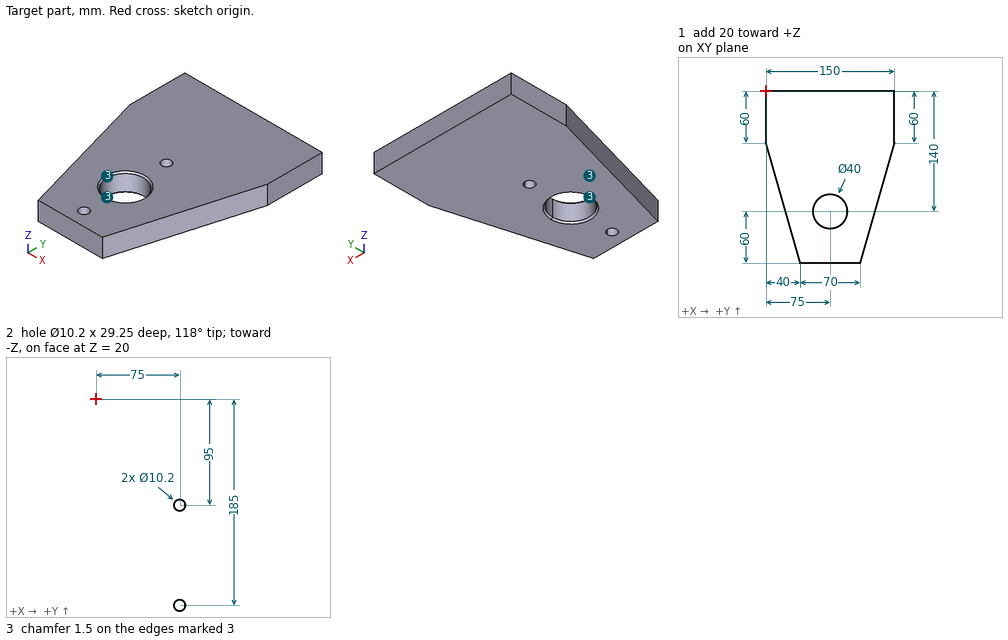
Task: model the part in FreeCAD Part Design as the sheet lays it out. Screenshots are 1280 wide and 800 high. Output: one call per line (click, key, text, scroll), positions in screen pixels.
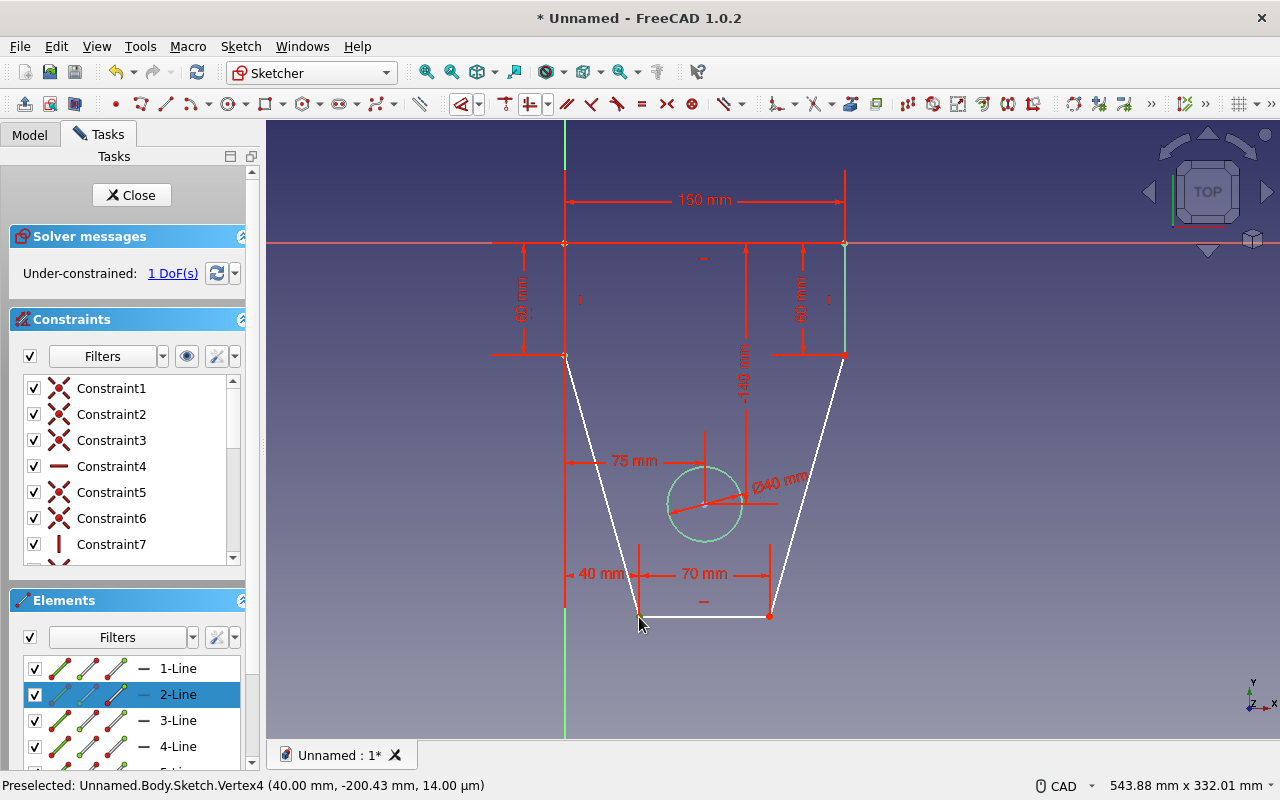
click(705, 504)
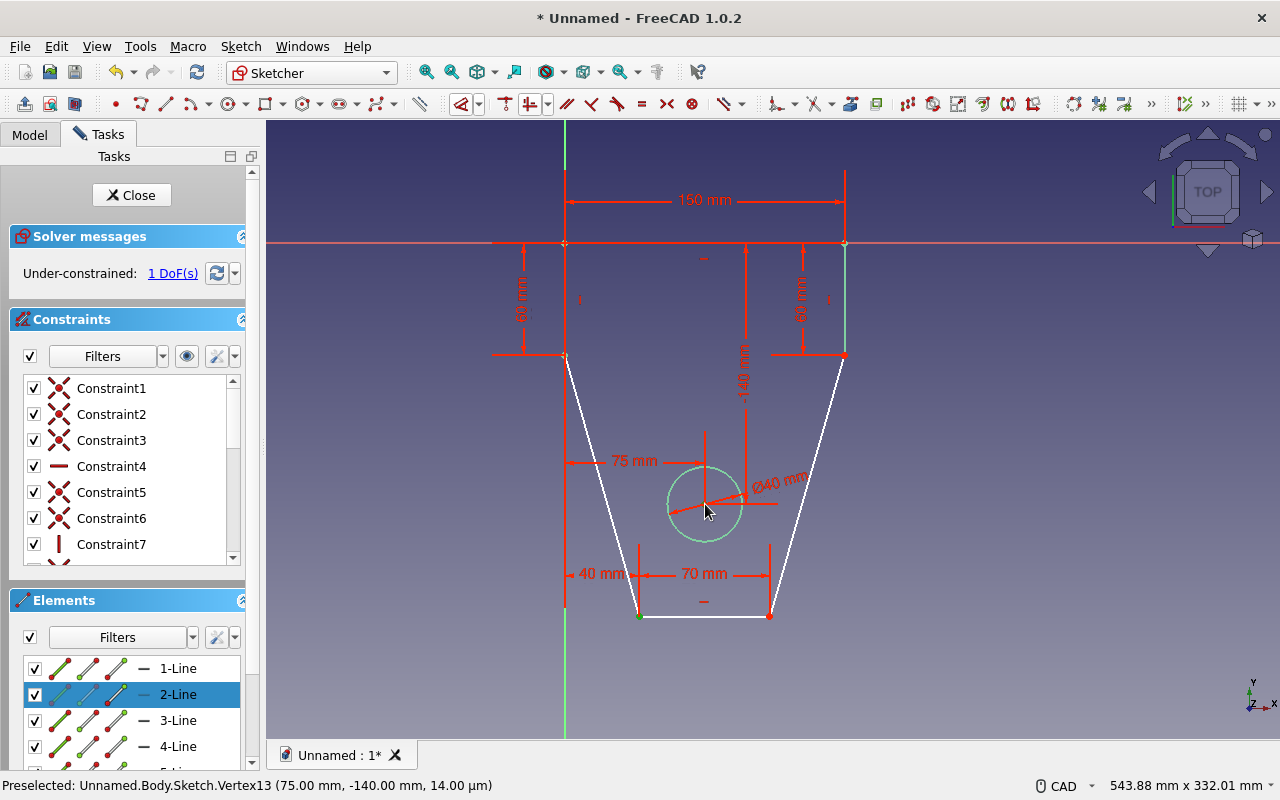
click(478, 104)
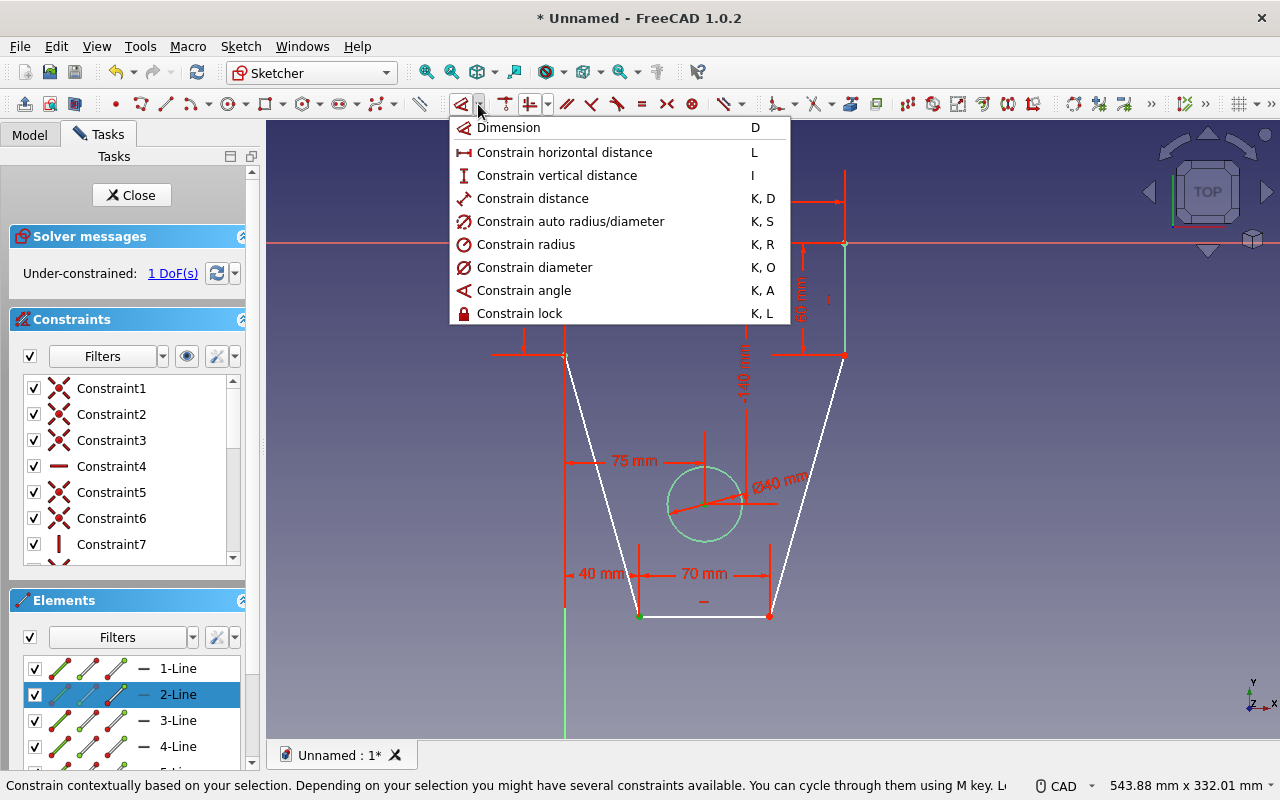
click(620, 176)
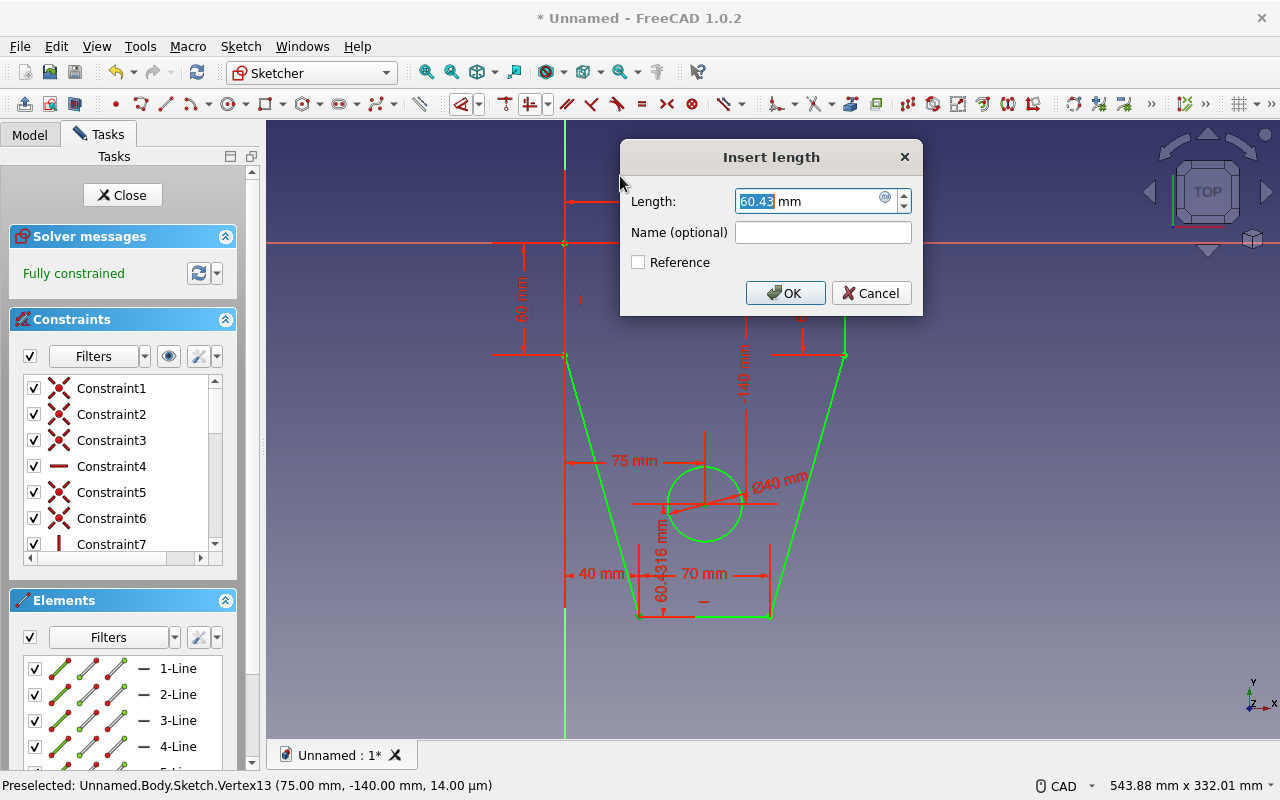
text(60)
key(Return)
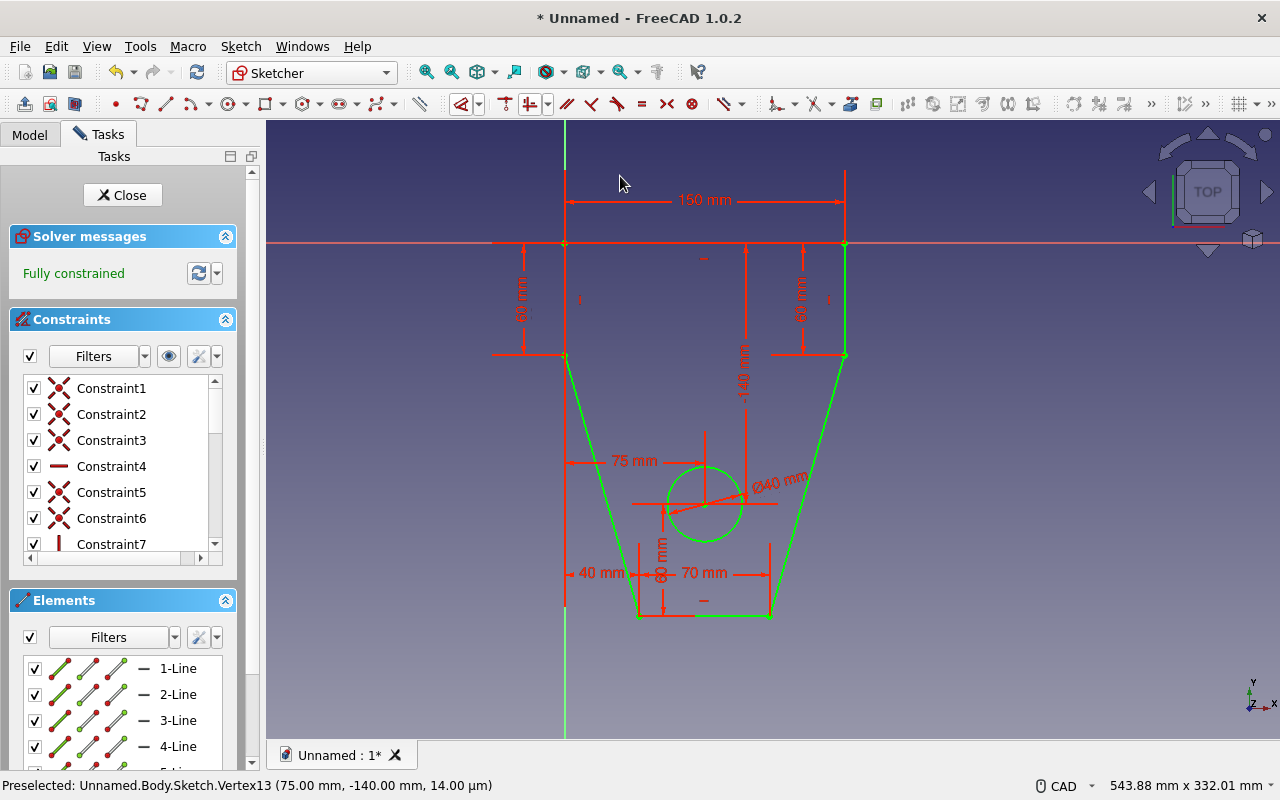
click(123, 195)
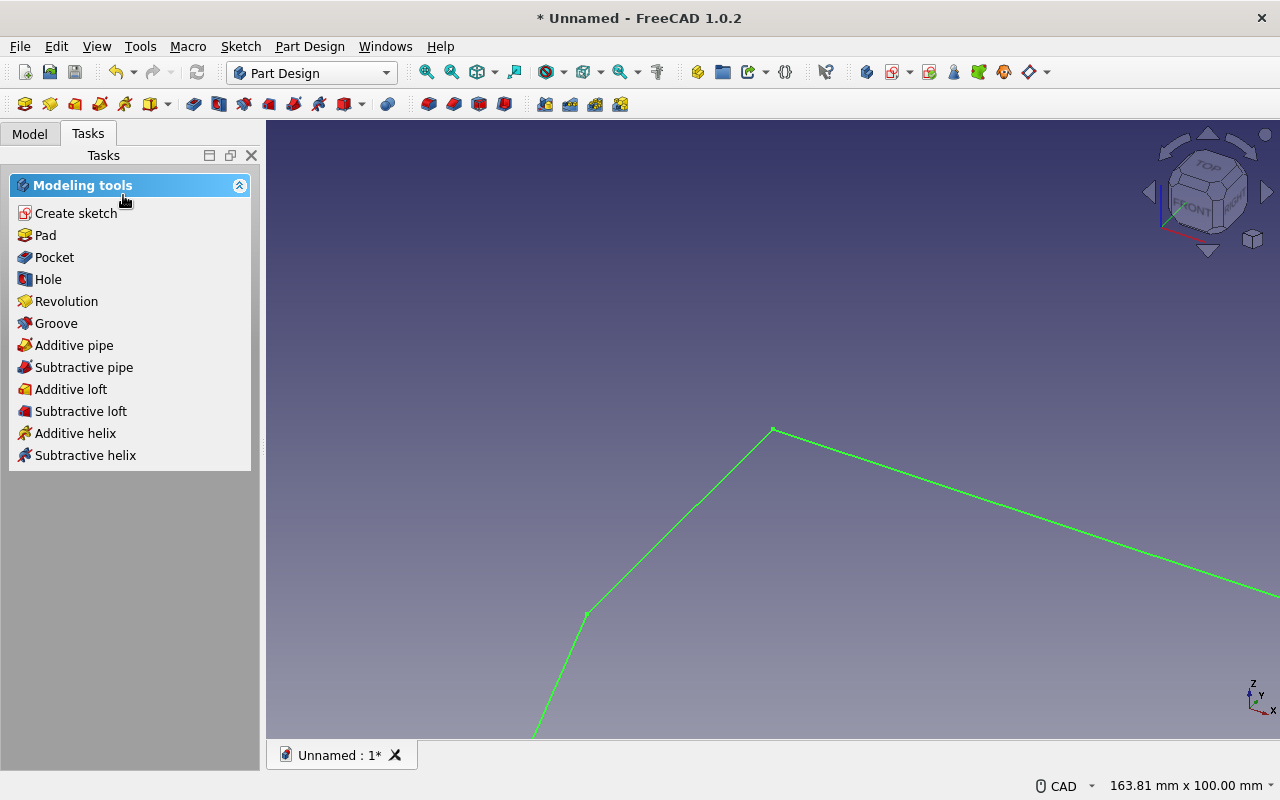
click(25, 104)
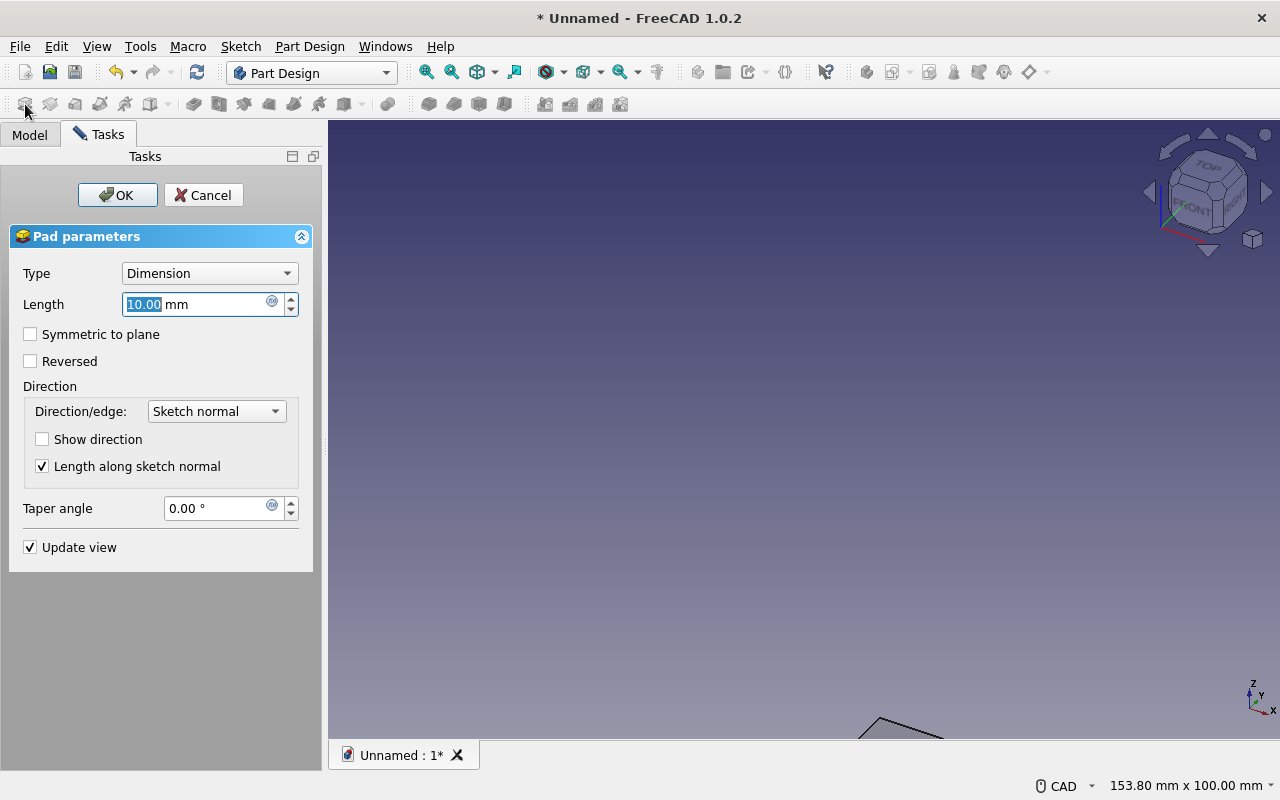
text(20)
key(Tab)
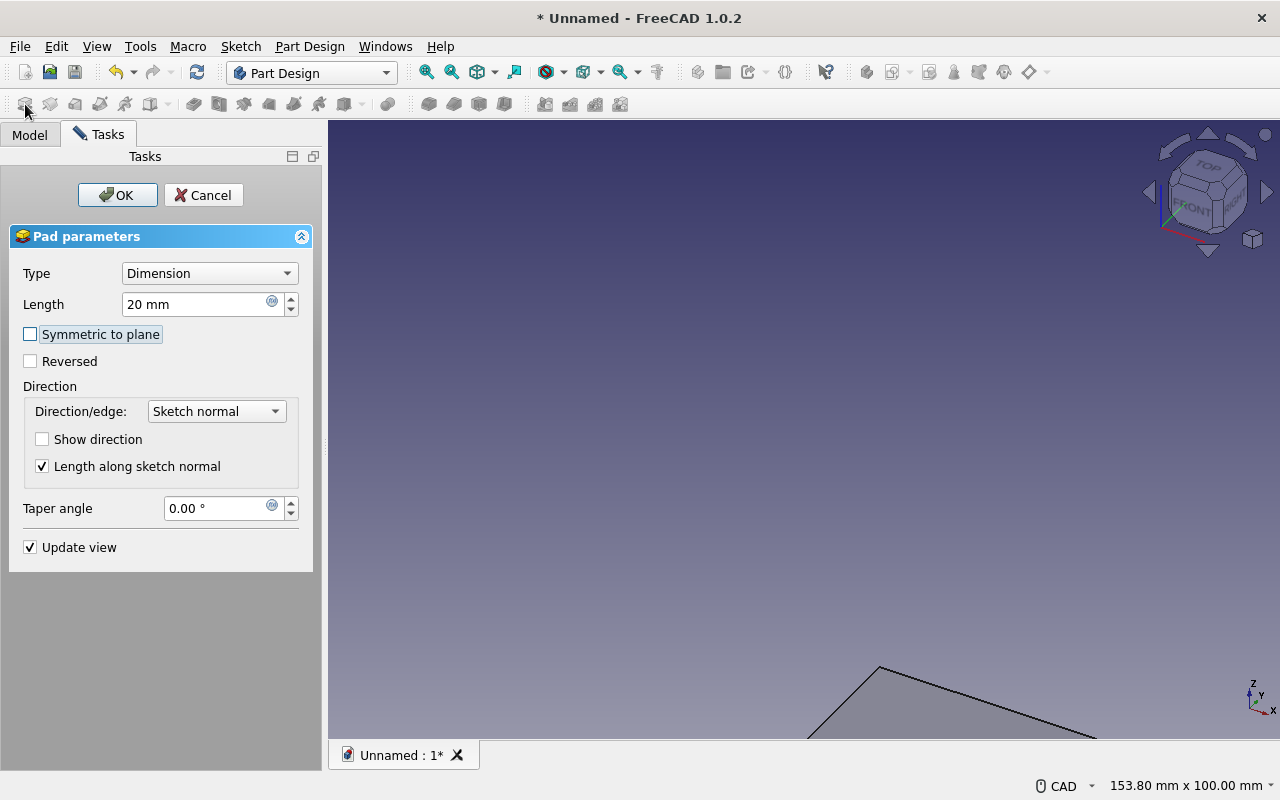
click(118, 195)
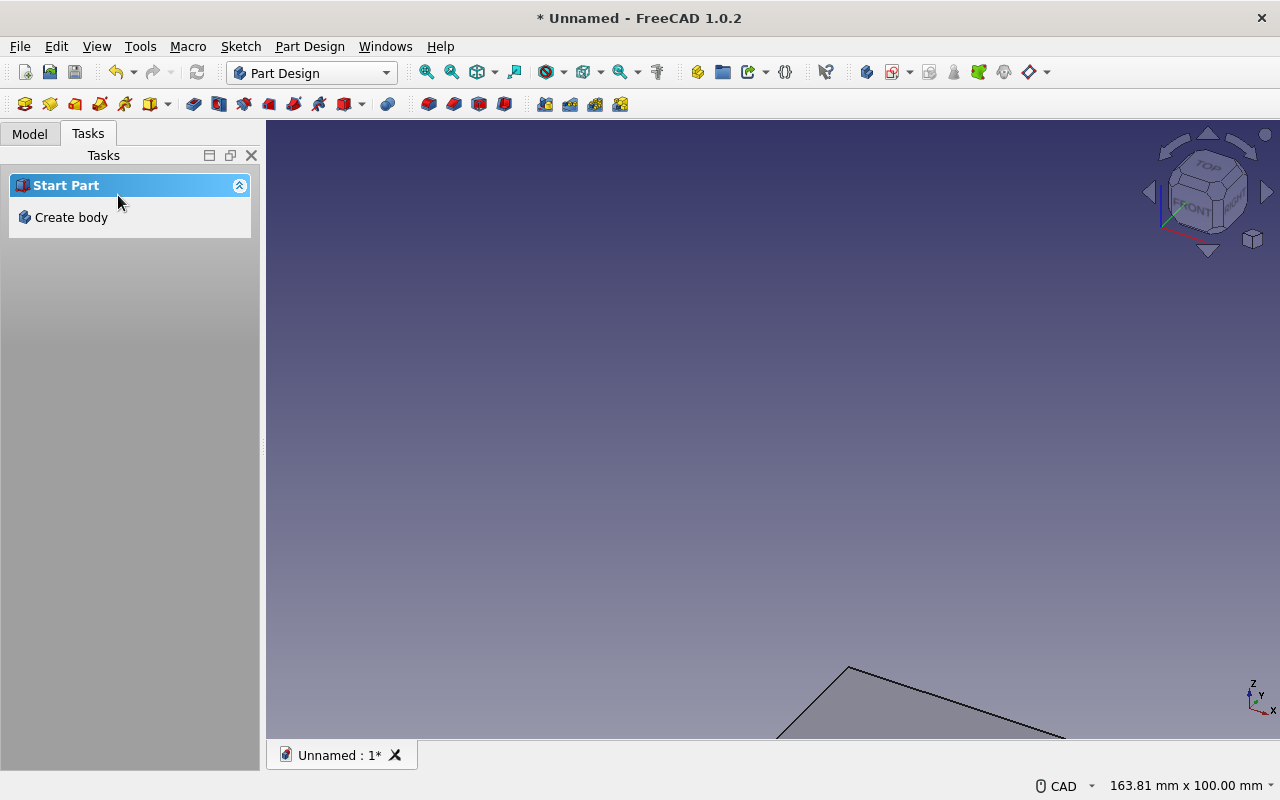
click(427, 72)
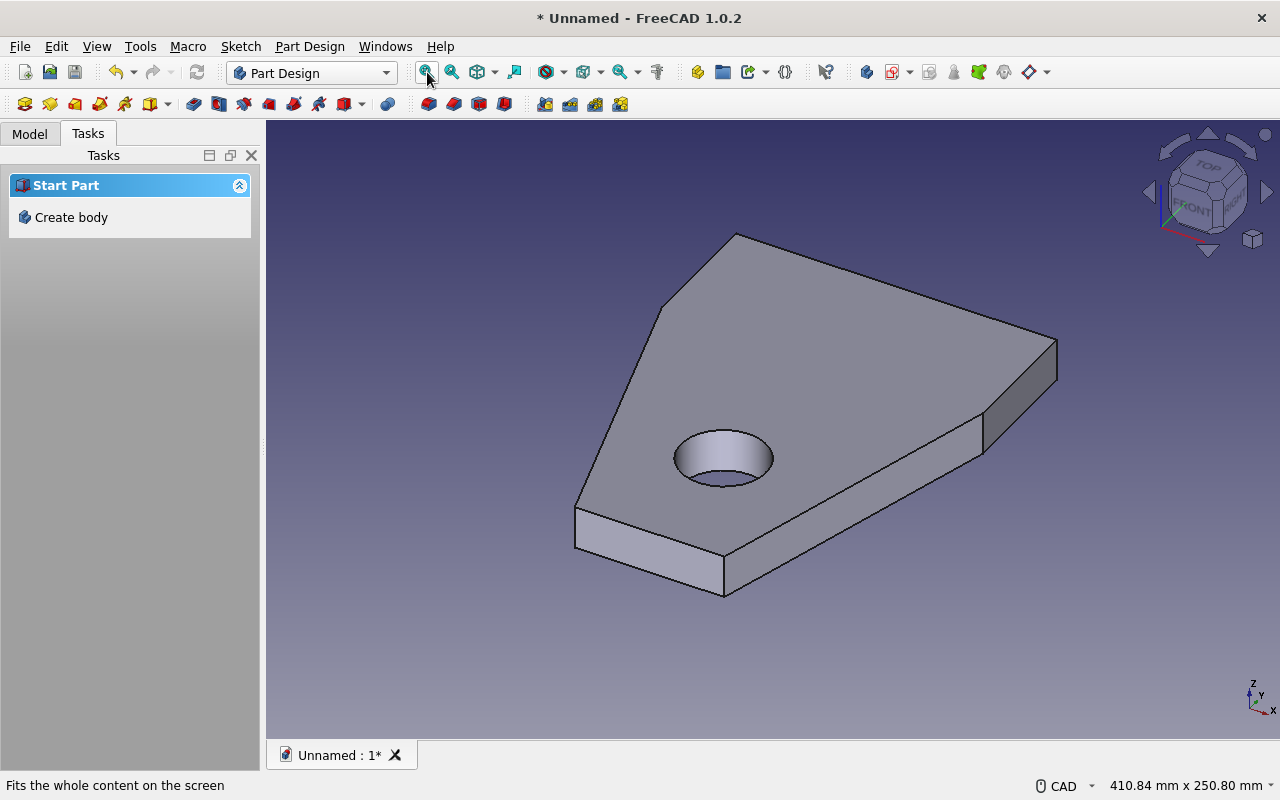
click(808, 373)